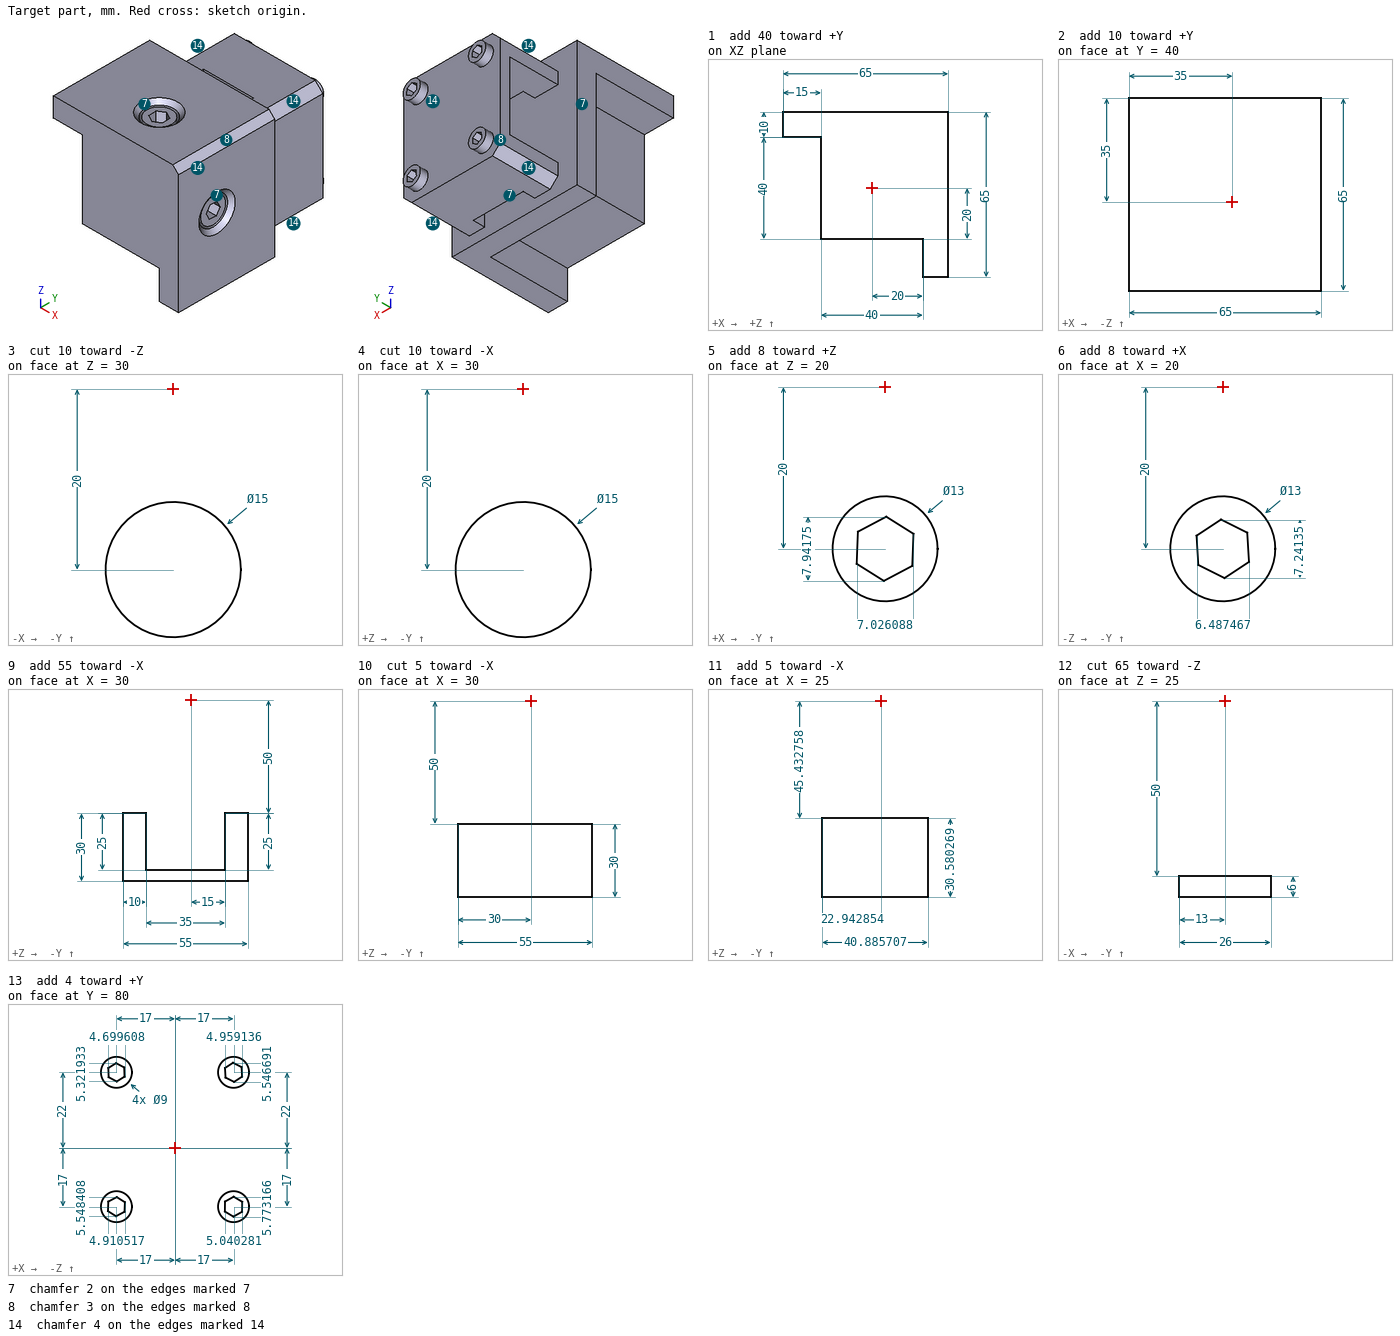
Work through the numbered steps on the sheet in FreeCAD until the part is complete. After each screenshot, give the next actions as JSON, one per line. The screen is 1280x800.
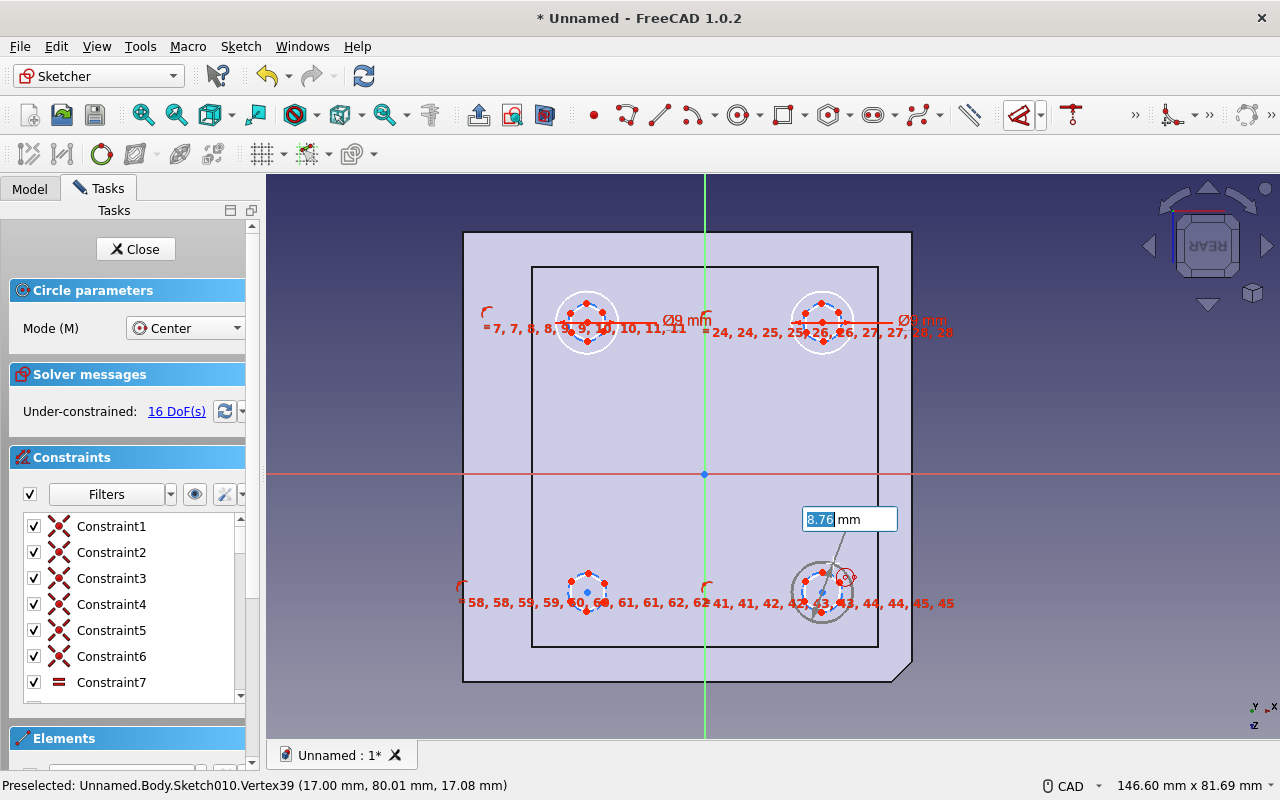
{"action": "type", "text": "9"}
{"action": "key", "text": "Return"}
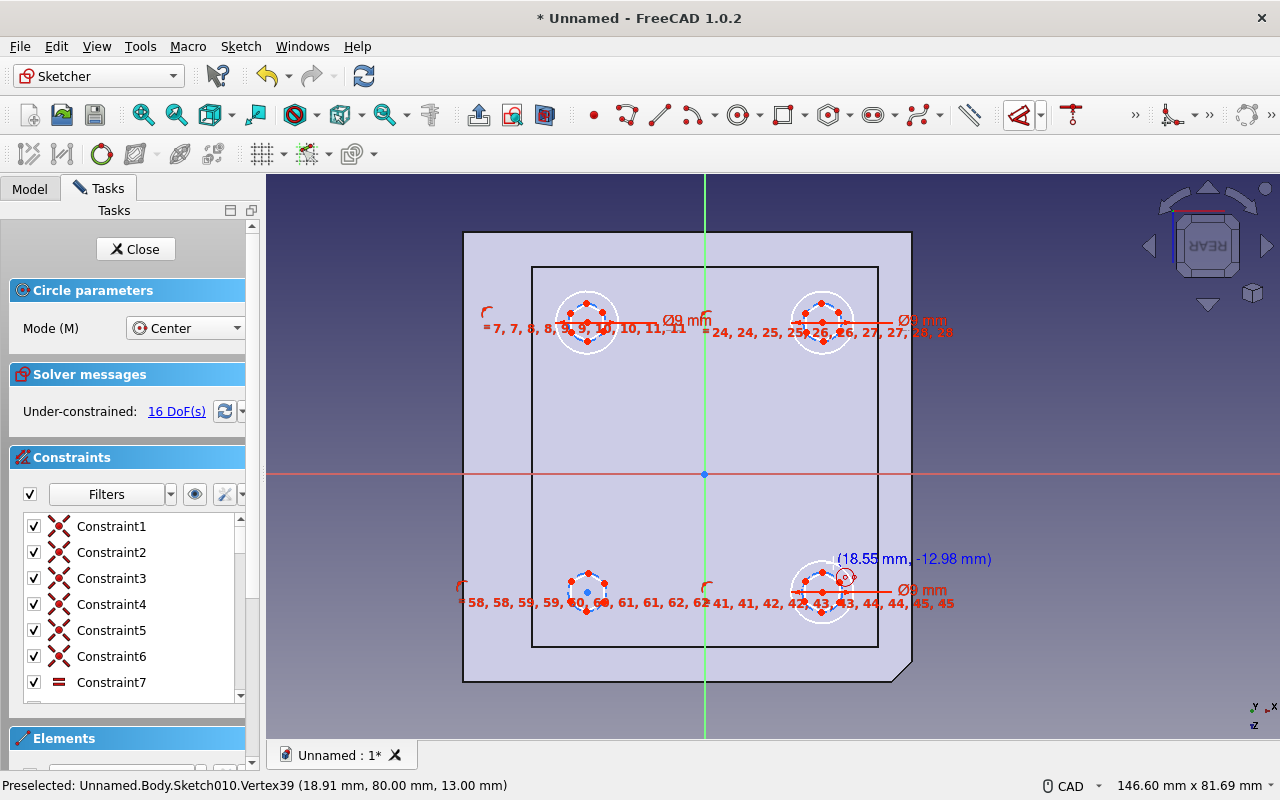
{"action": "left_click", "coordinate": [587, 592]}
{"action": "mouse_move", "coordinate": [598, 563]}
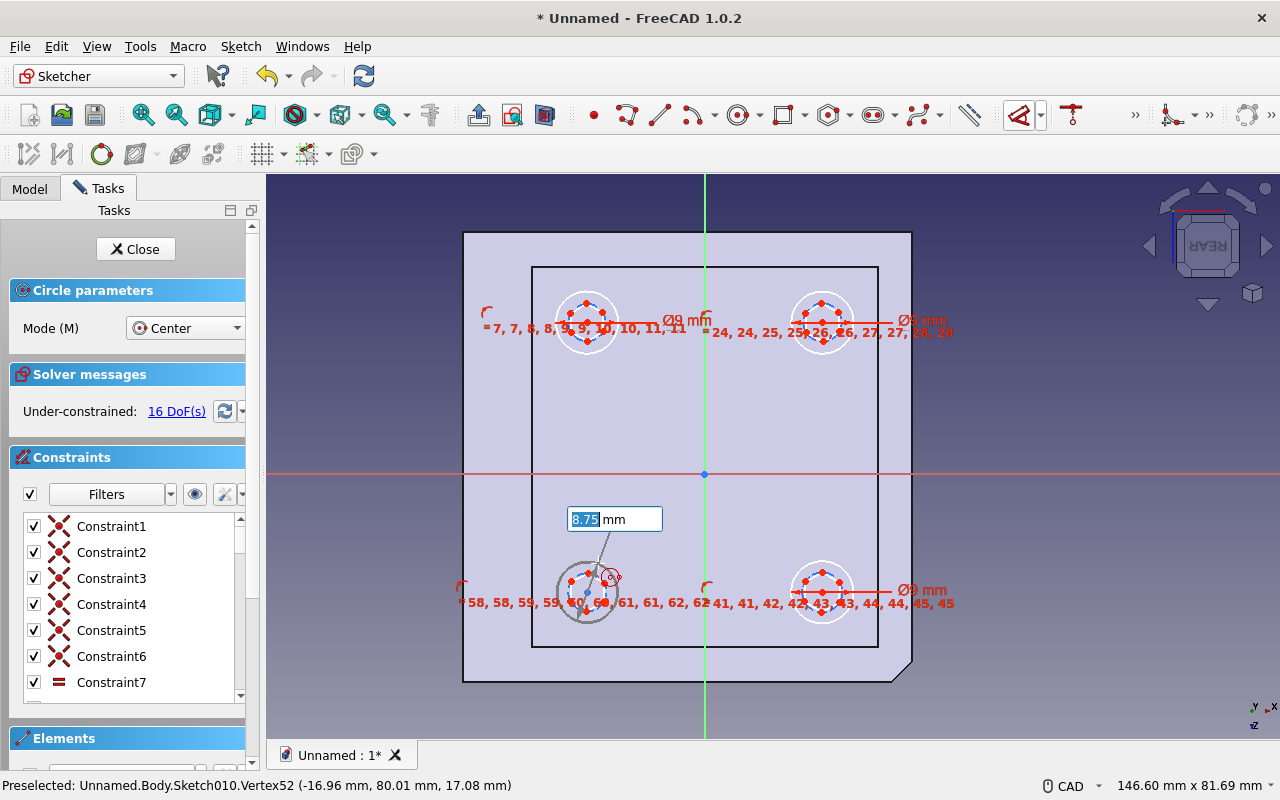
{"action": "type", "text": "9"}
{"action": "key", "text": "Return"}
{"action": "key", "text": "Escape"}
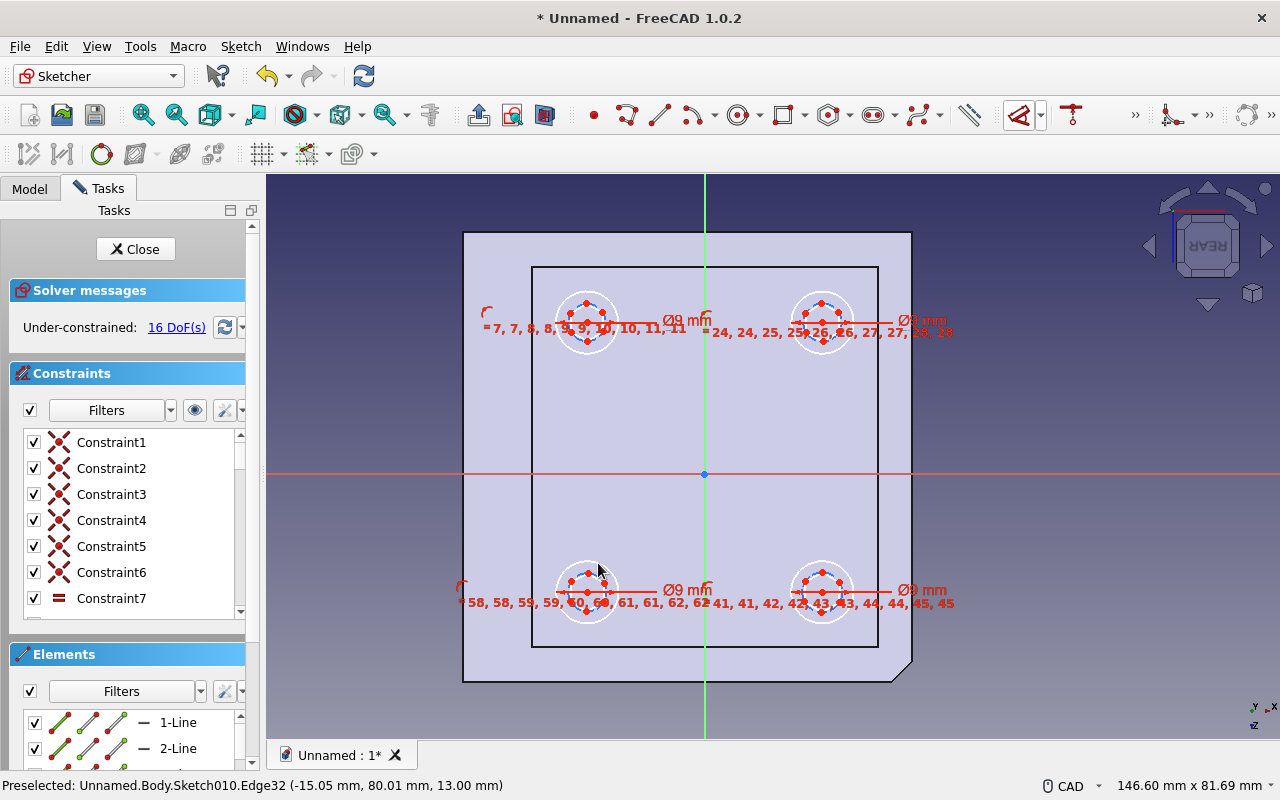
{"action": "left_click", "coordinate": [587, 323]}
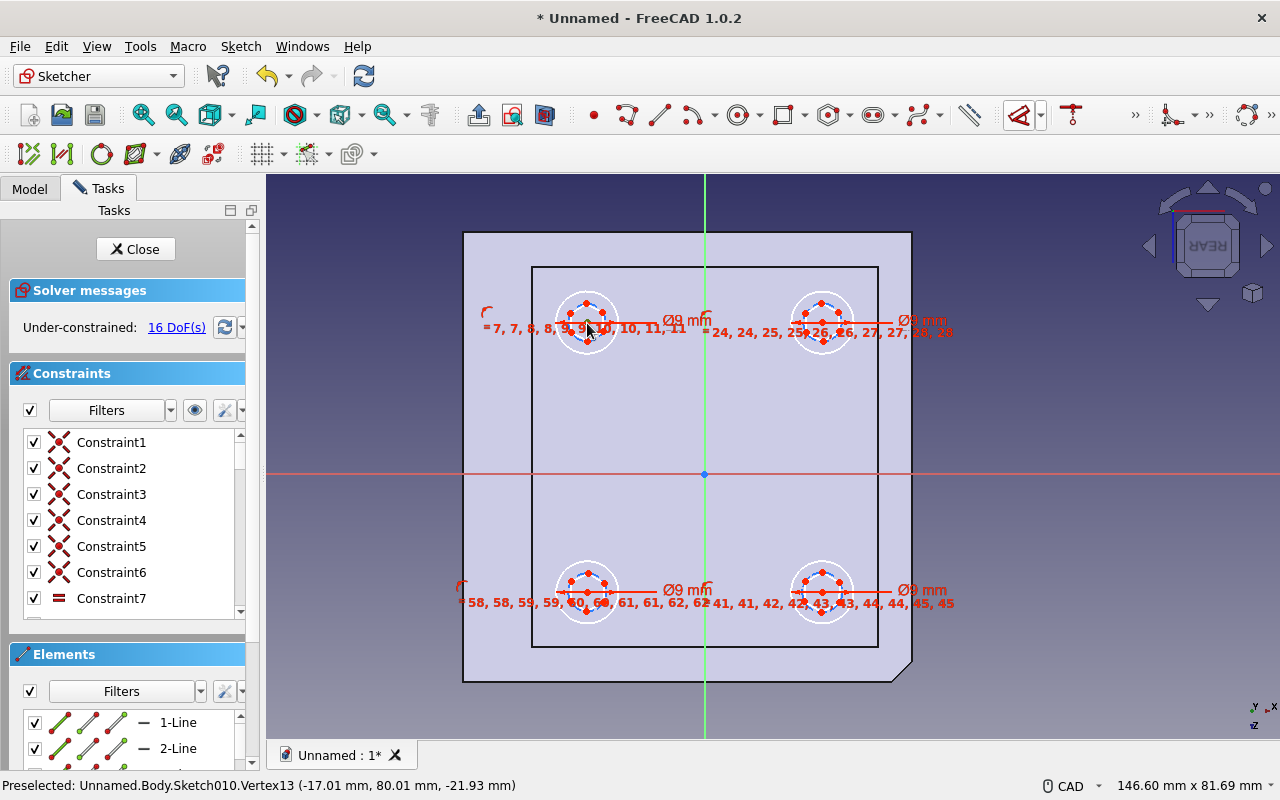
{"action": "key", "text": "l"}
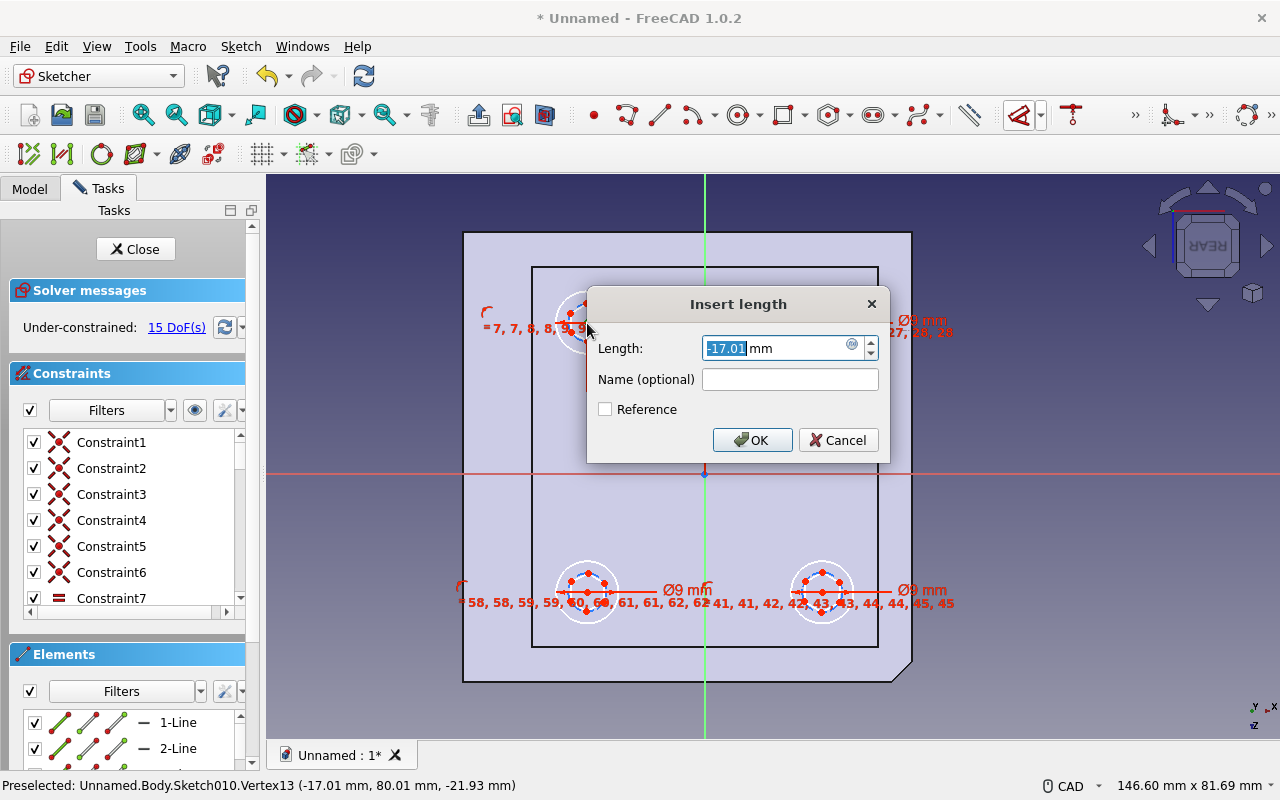
{"action": "type", "text": "-17"}
{"action": "key", "text": "Return"}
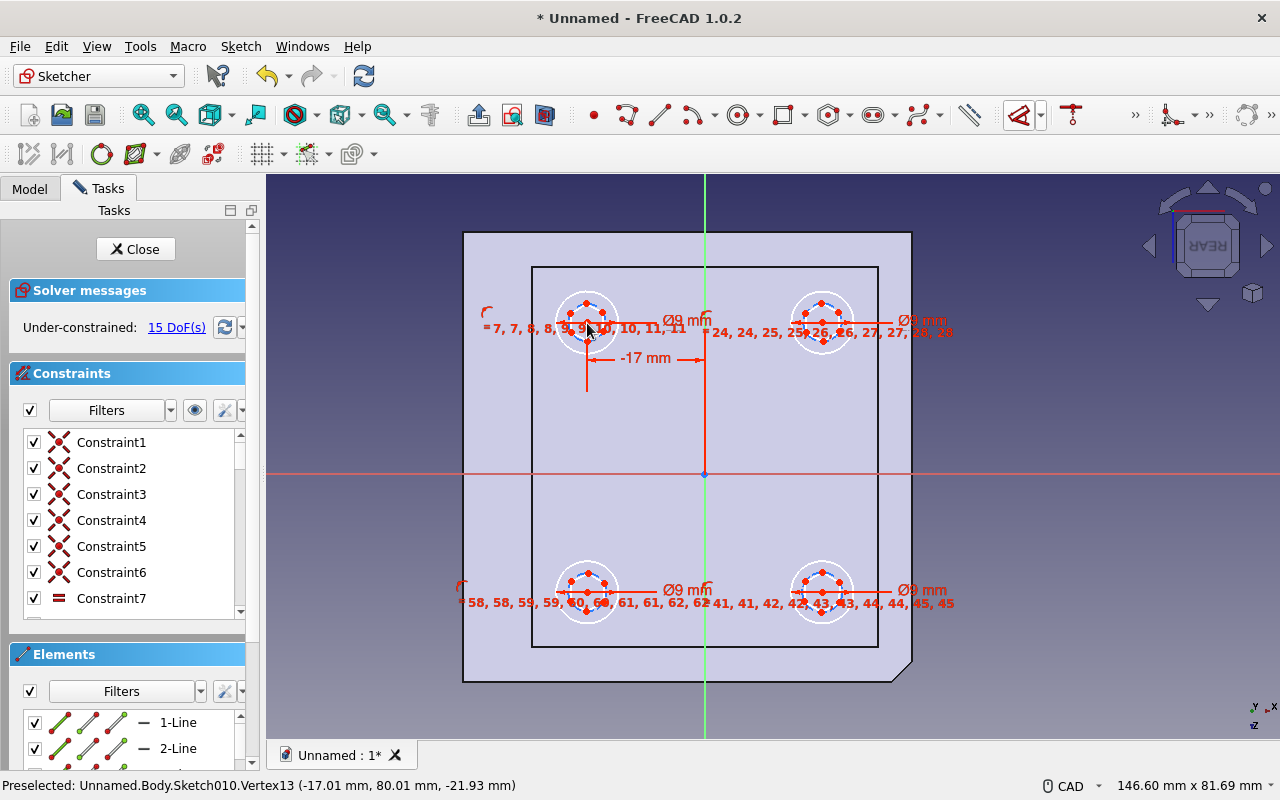
{"action": "left_click", "coordinate": [587, 323]}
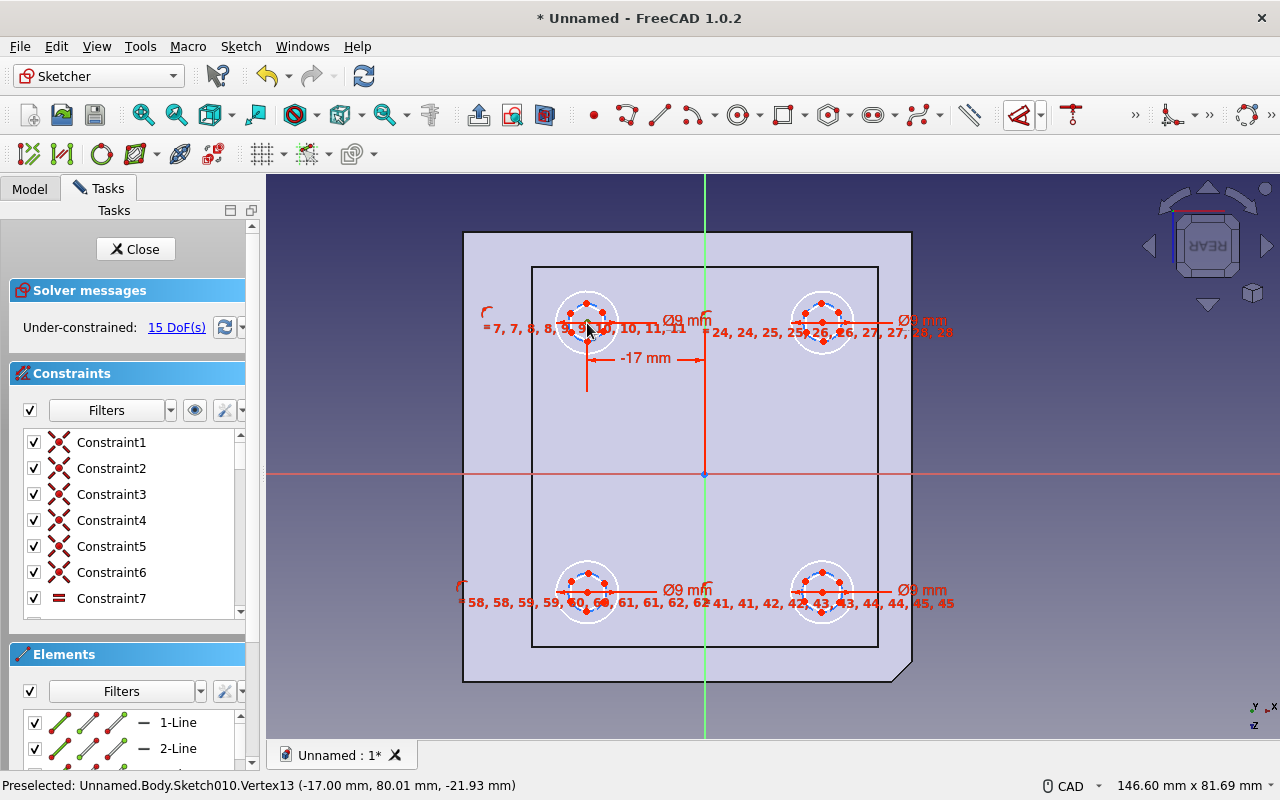
{"action": "left_click", "coordinate": [1040, 116]}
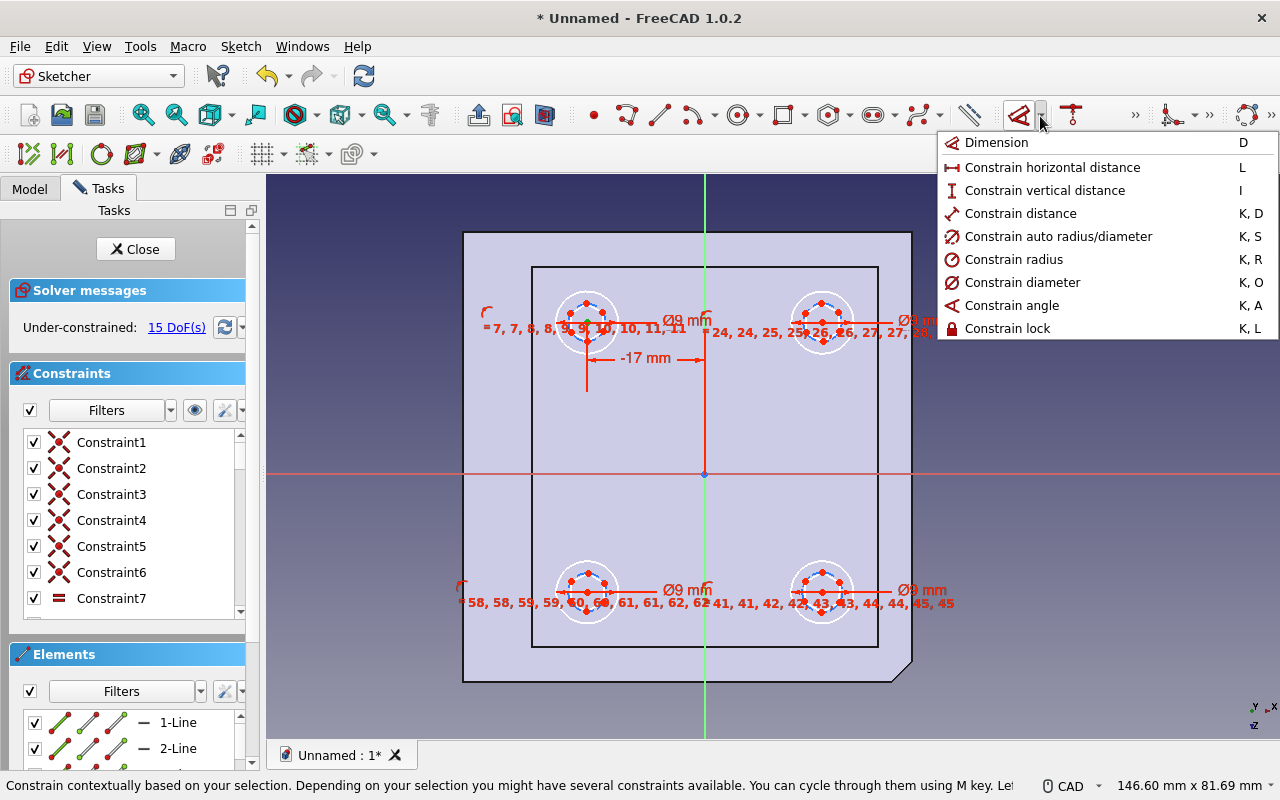
{"action": "left_click", "coordinate": [1108, 190]}